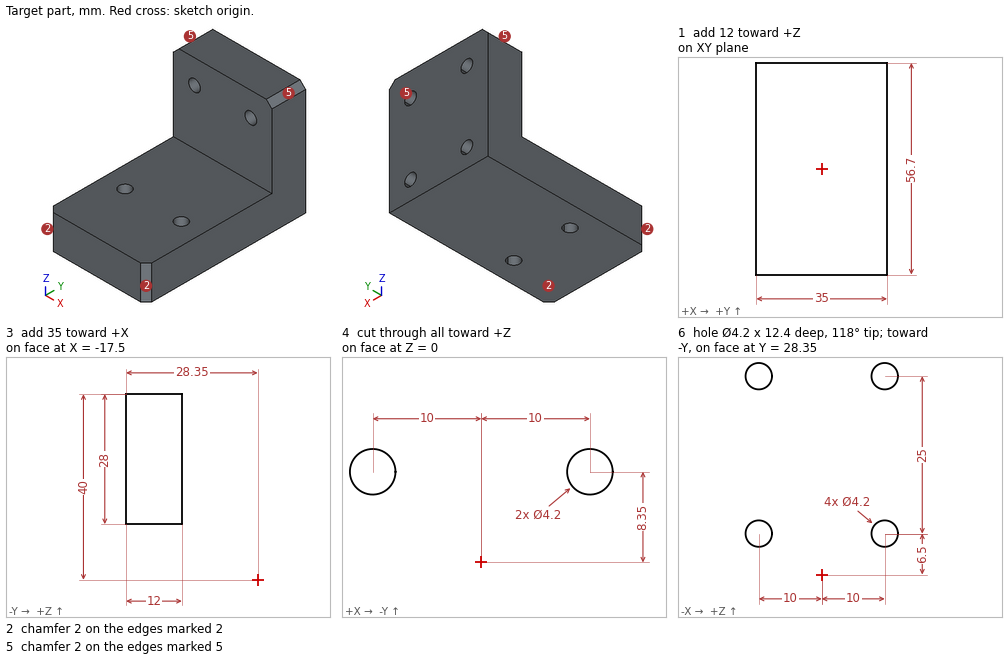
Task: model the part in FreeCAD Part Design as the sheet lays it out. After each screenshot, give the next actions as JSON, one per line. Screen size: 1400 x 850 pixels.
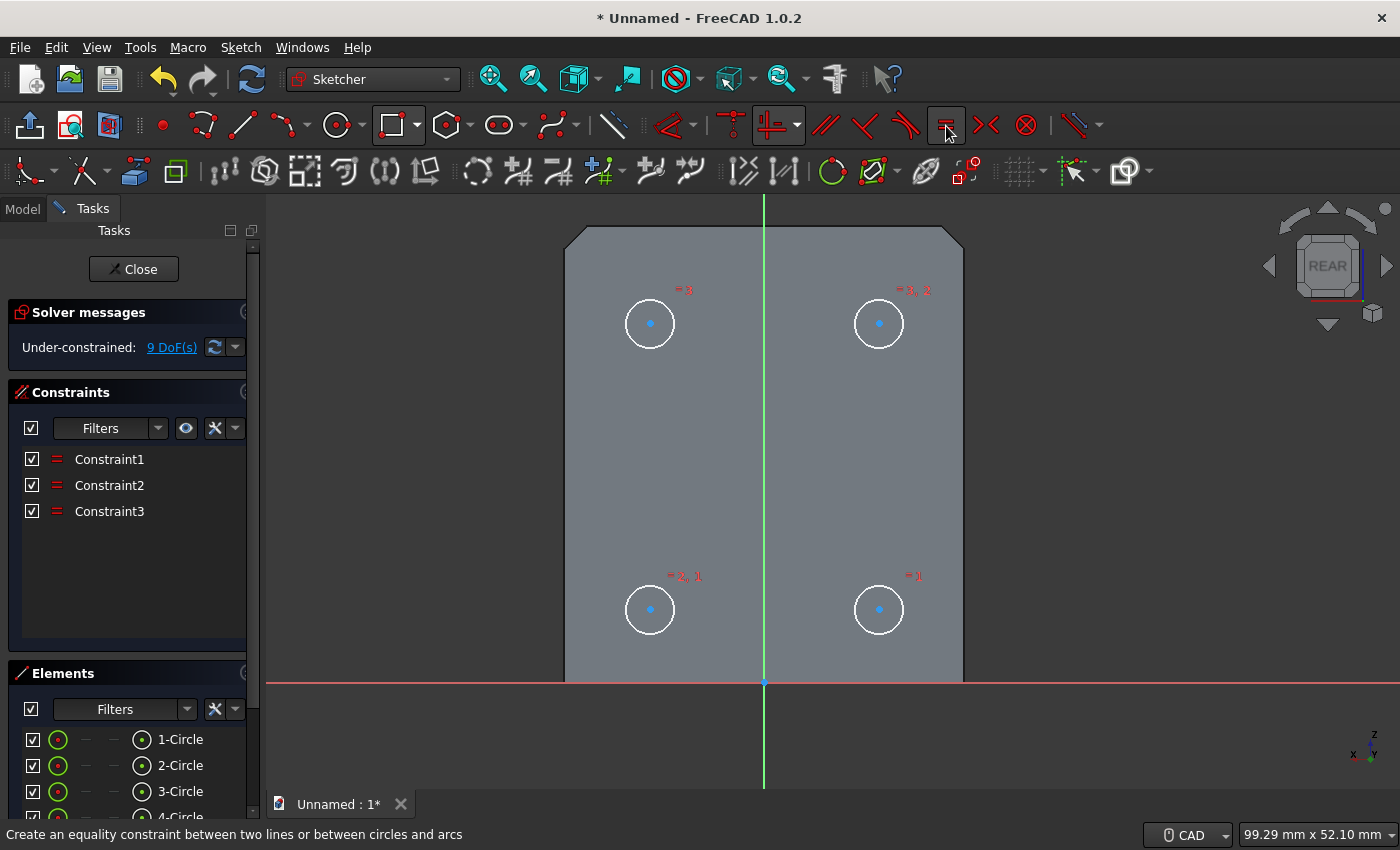
{"action": "left_click", "coordinate": [879, 610]}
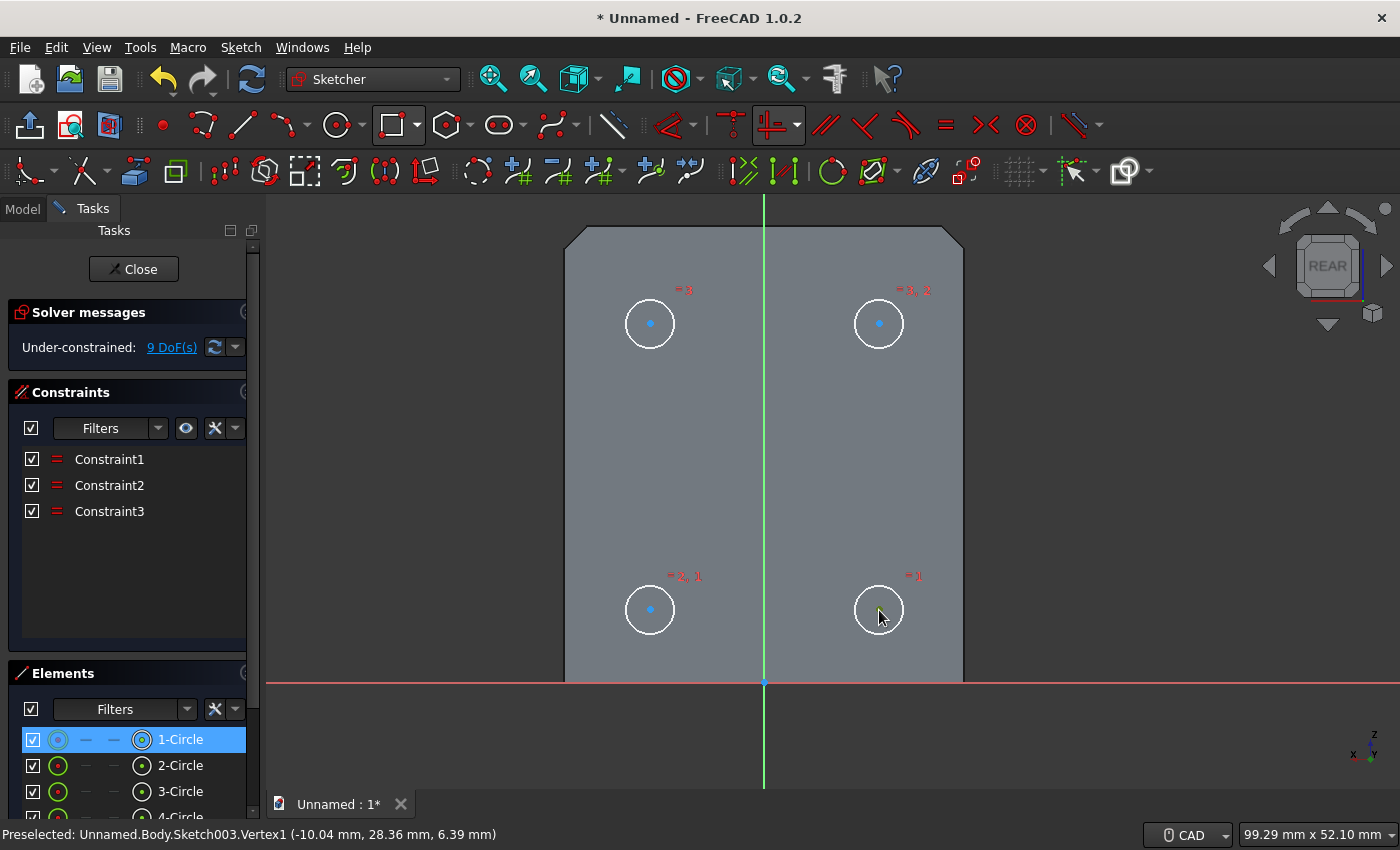
{"action": "left_click", "coordinate": [650, 610]}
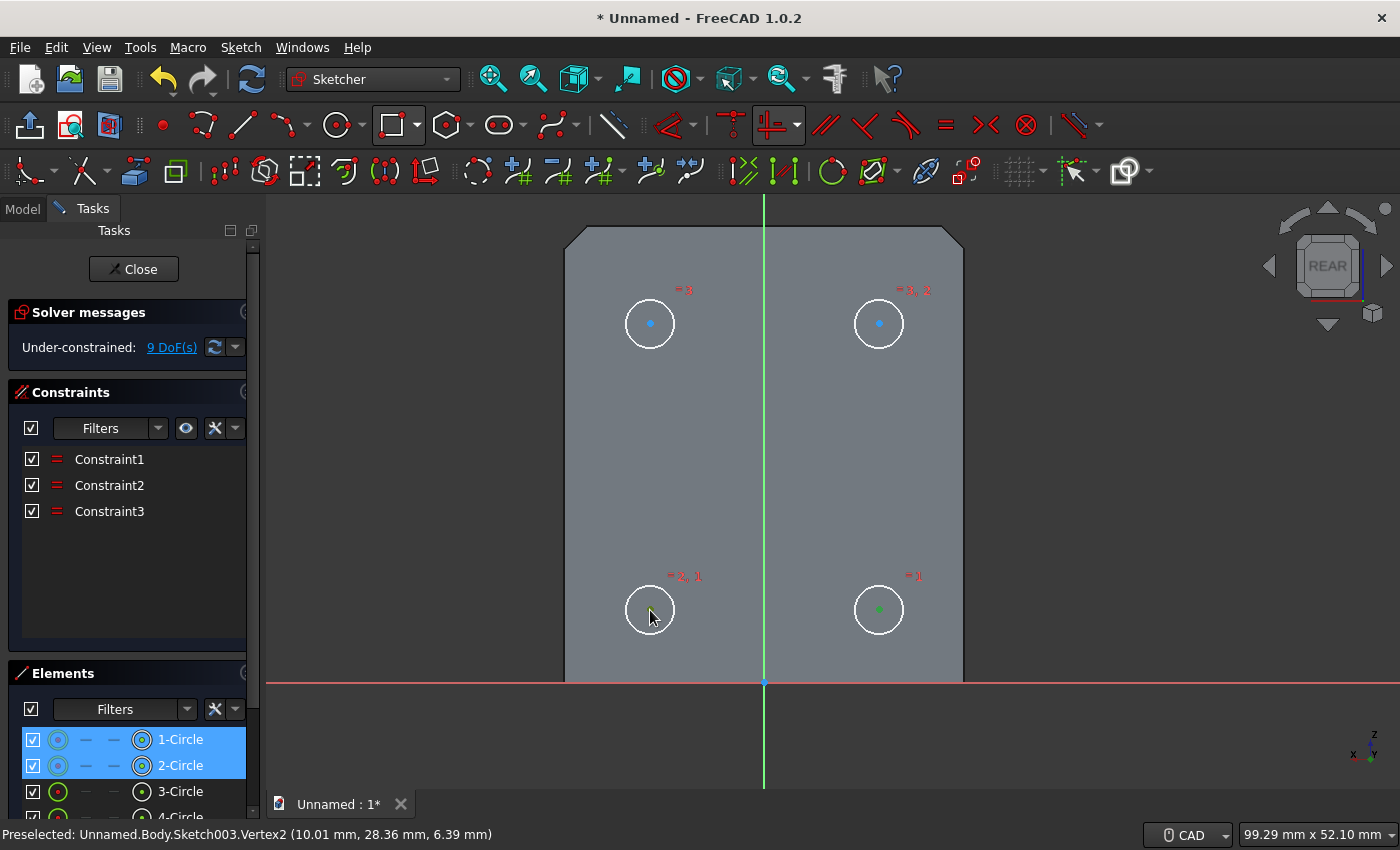
{"action": "left_click", "coordinate": [800, 126]}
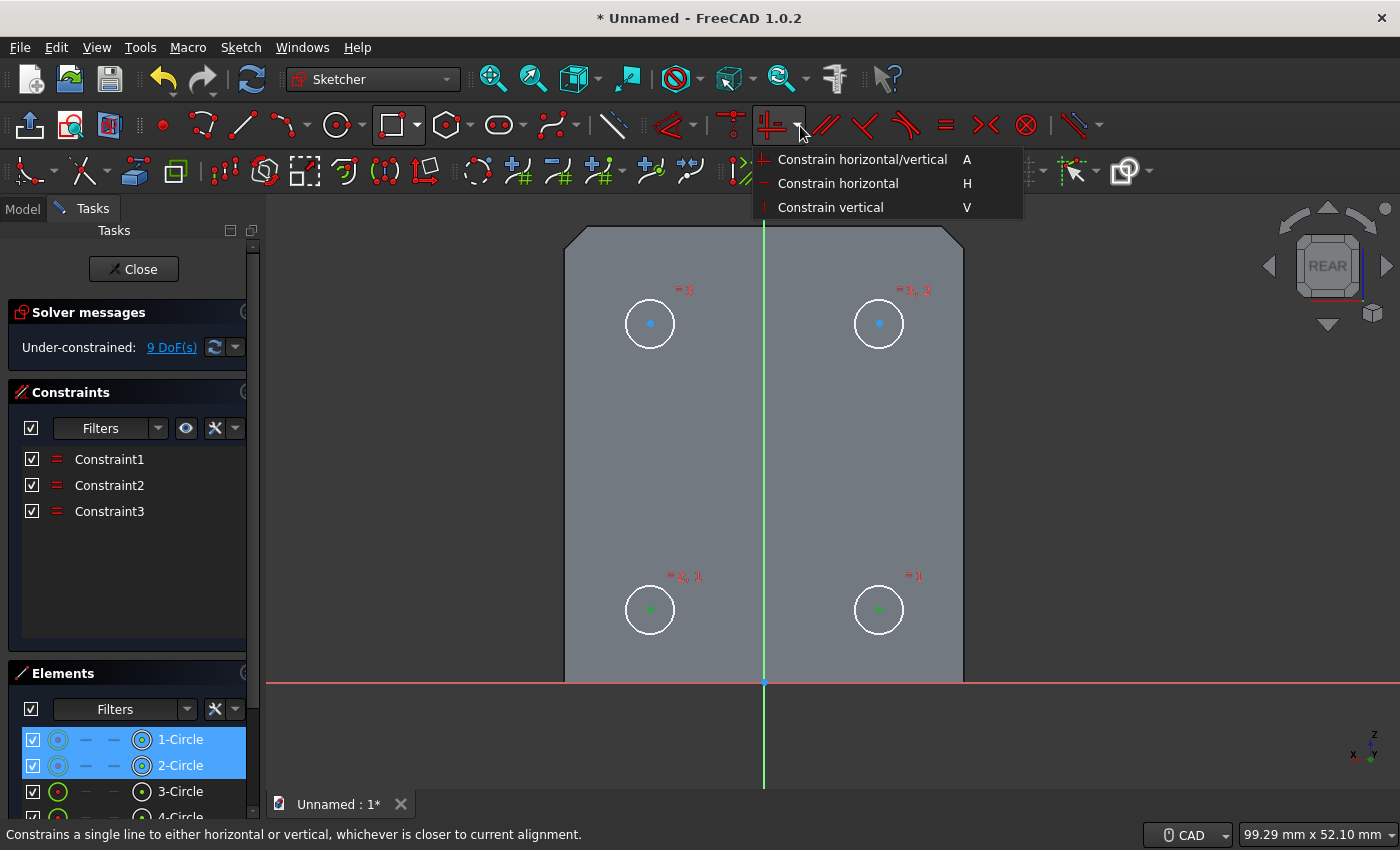
{"action": "left_click", "coordinate": [888, 183]}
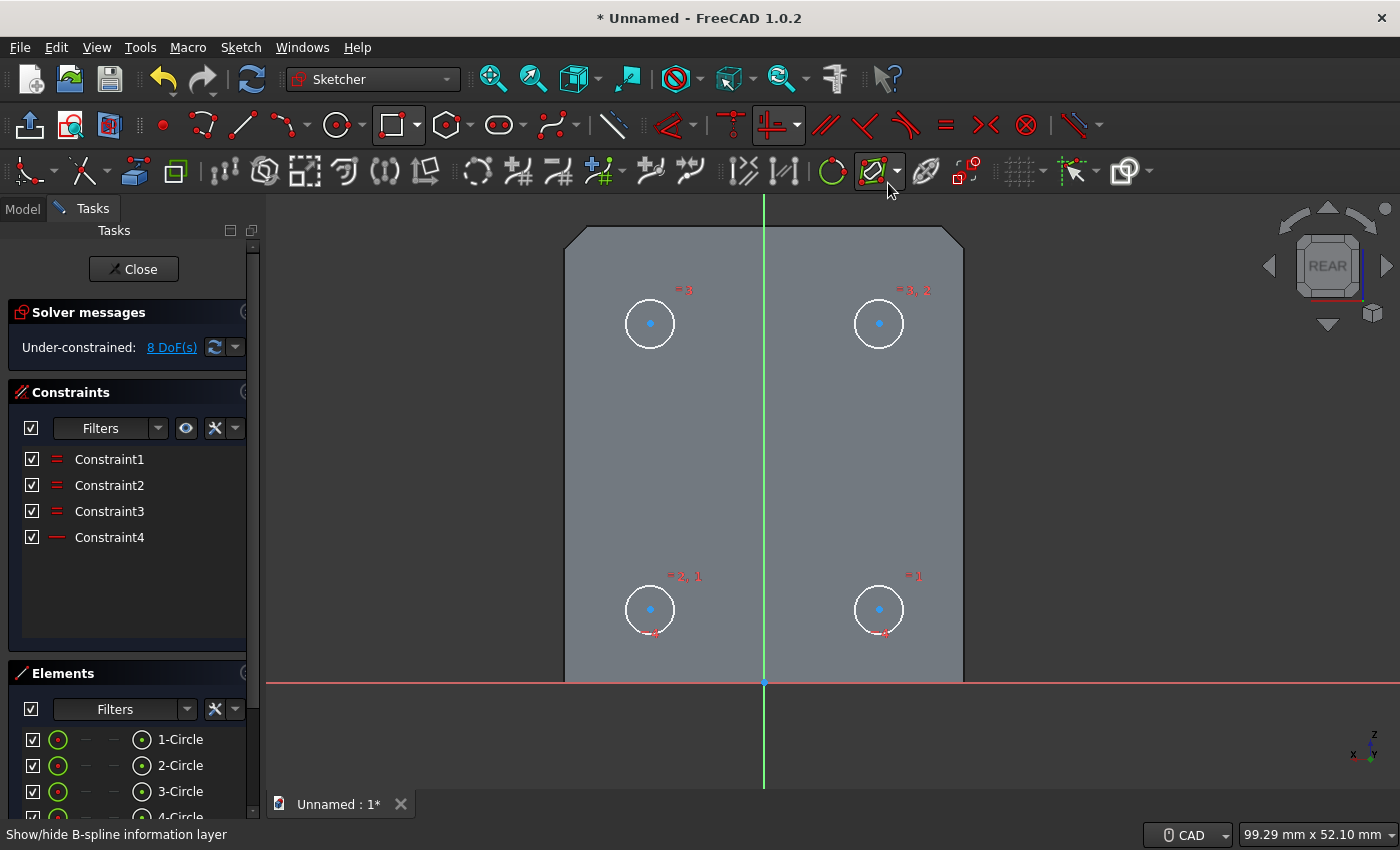
{"action": "left_click", "coordinate": [879, 610]}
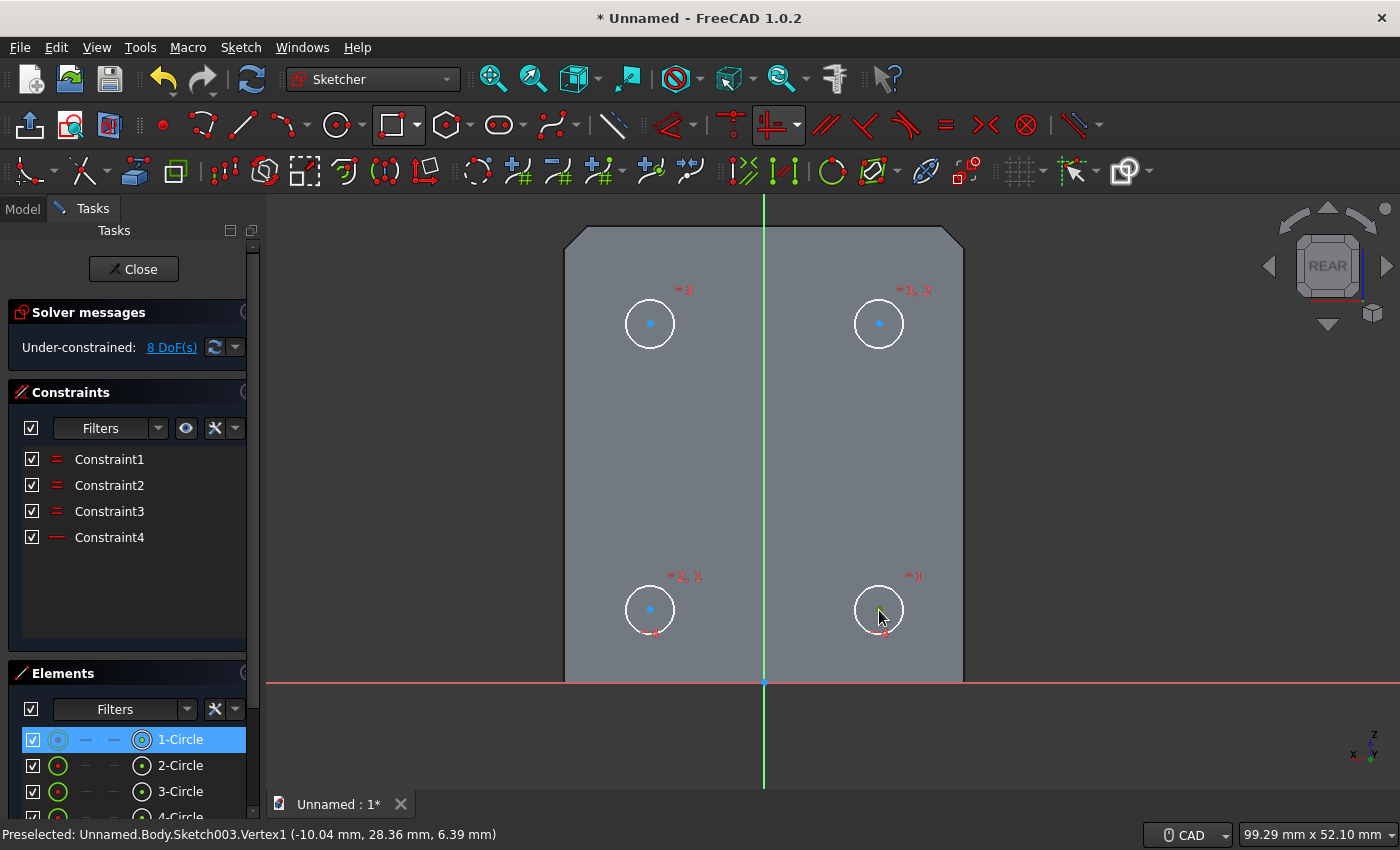
{"action": "left_click", "coordinate": [879, 324]}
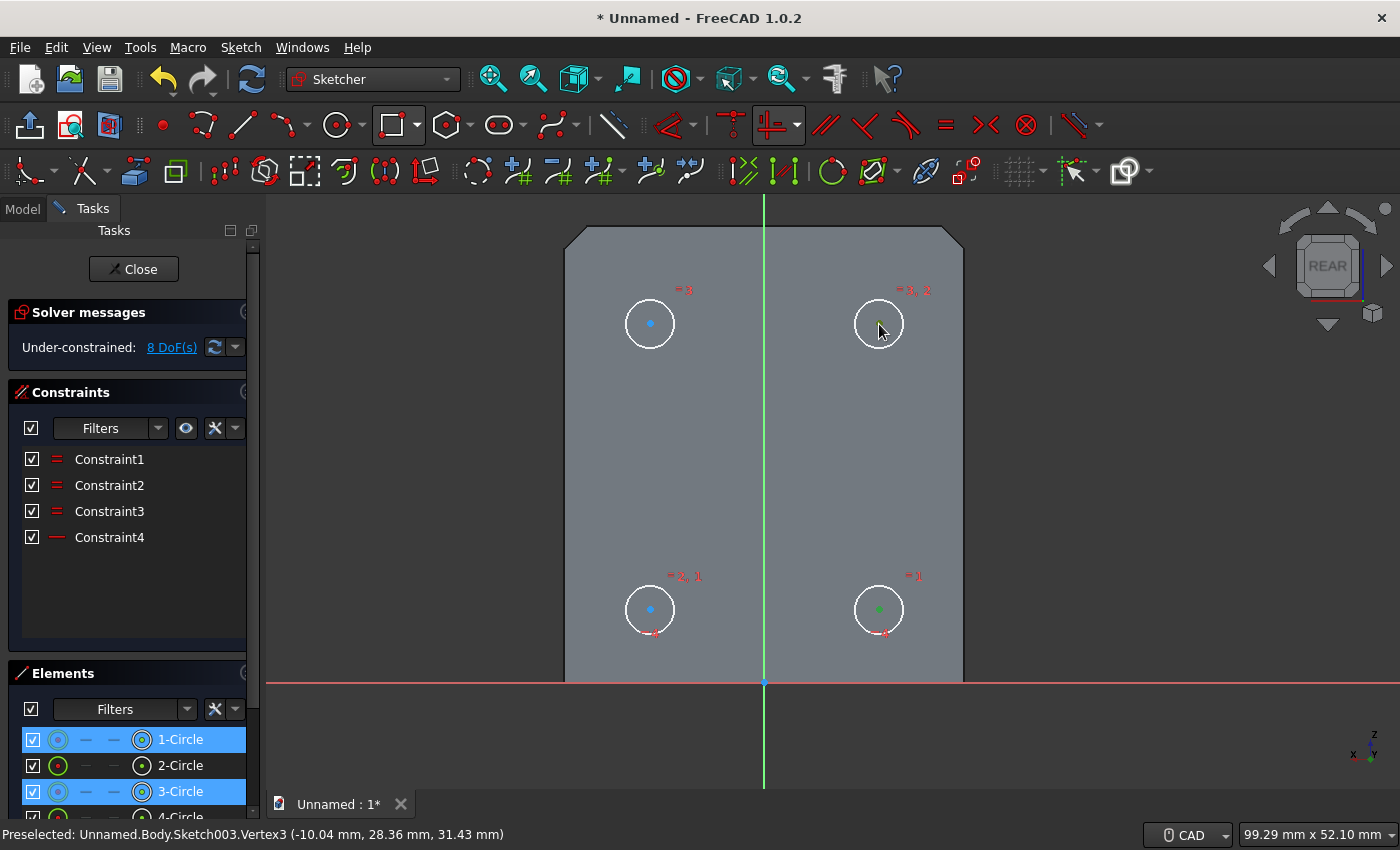
{"action": "key", "text": "v"}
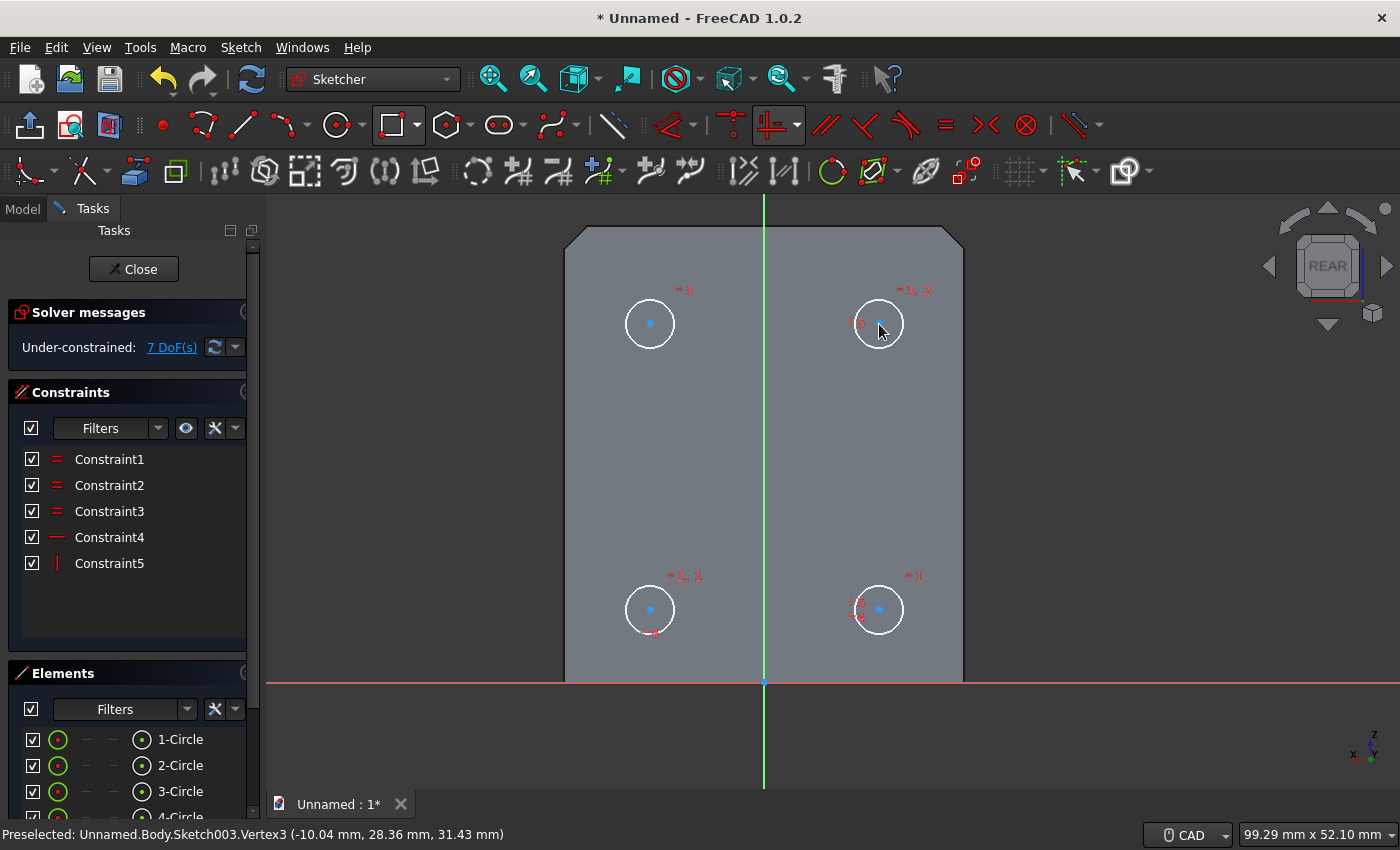
{"action": "left_click", "coordinate": [650, 610]}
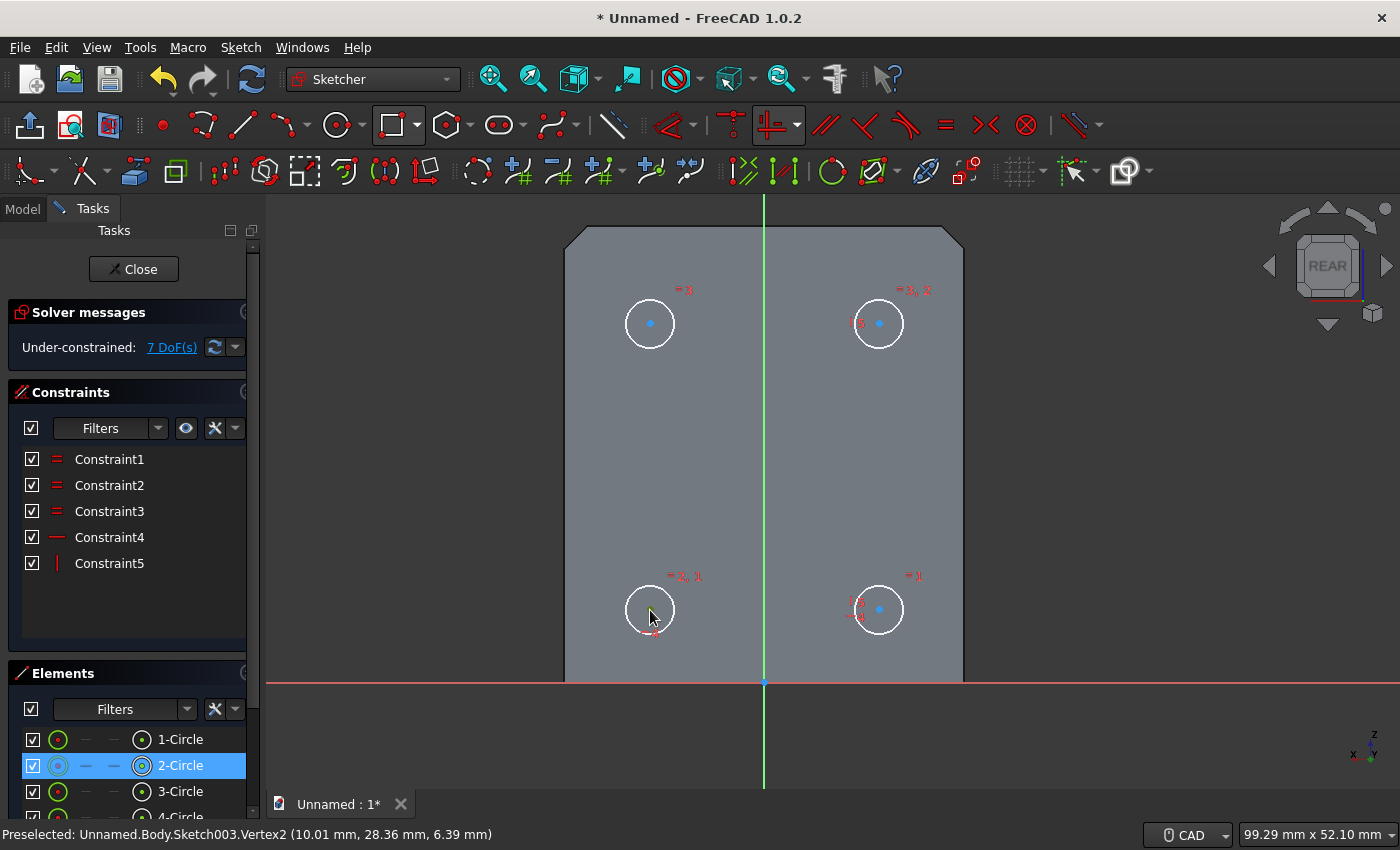
{"action": "left_click", "coordinate": [650, 324]}